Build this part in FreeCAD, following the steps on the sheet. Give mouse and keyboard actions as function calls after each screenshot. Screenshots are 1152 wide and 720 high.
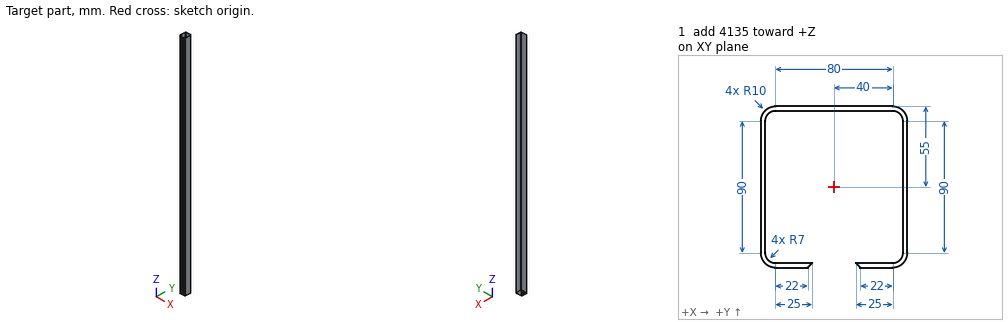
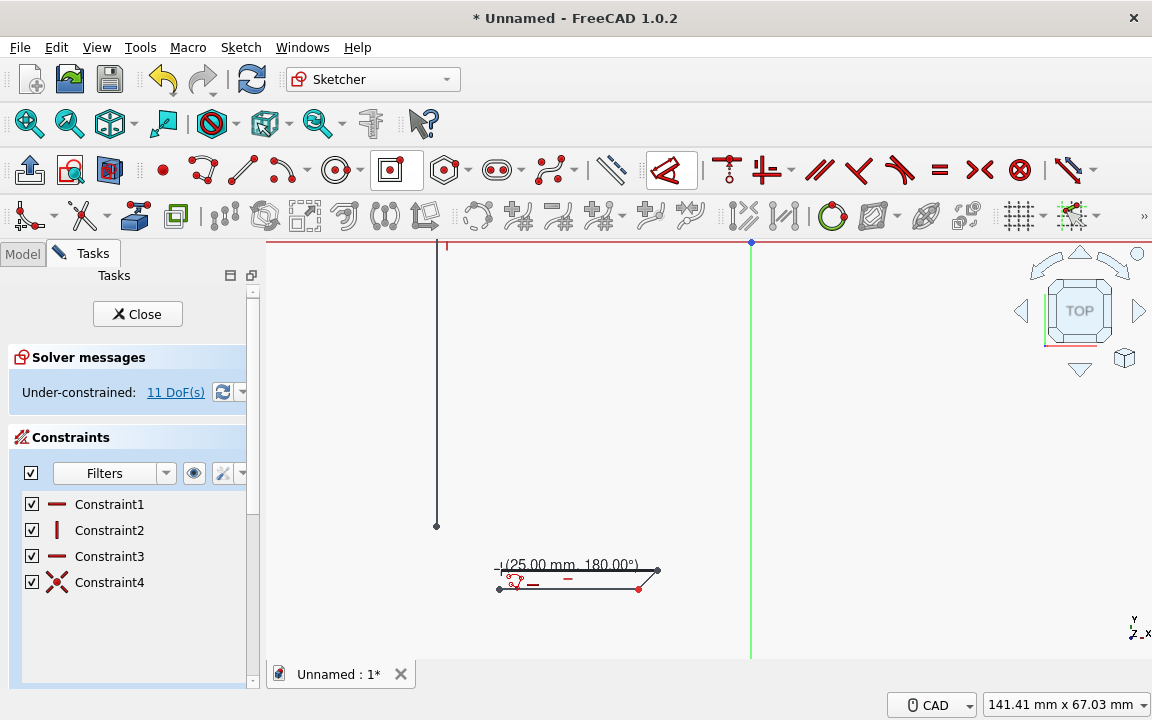
click(500, 569)
right_click(500, 569)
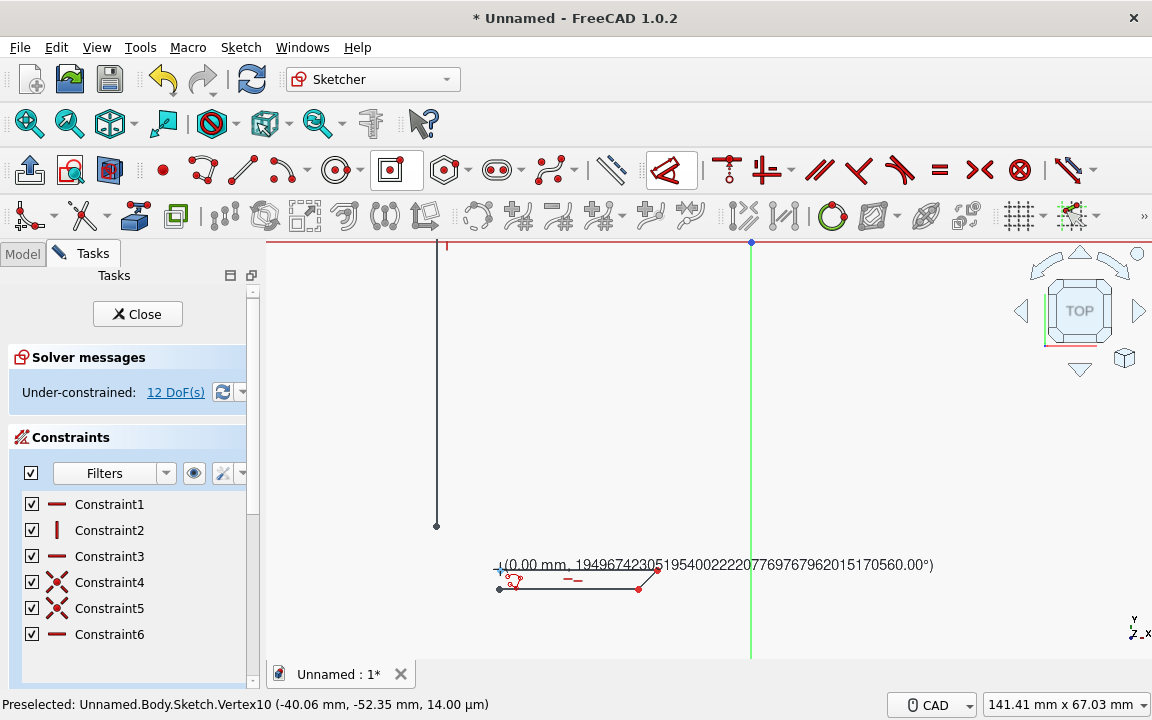
click(244, 170)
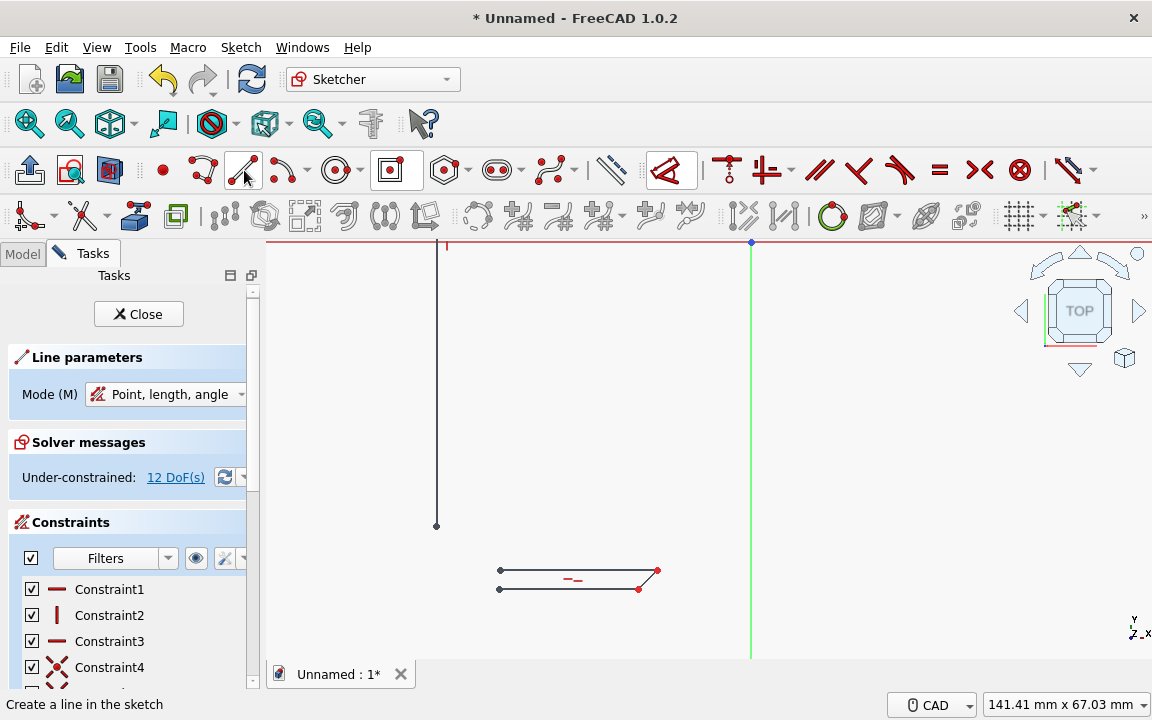
click(457, 524)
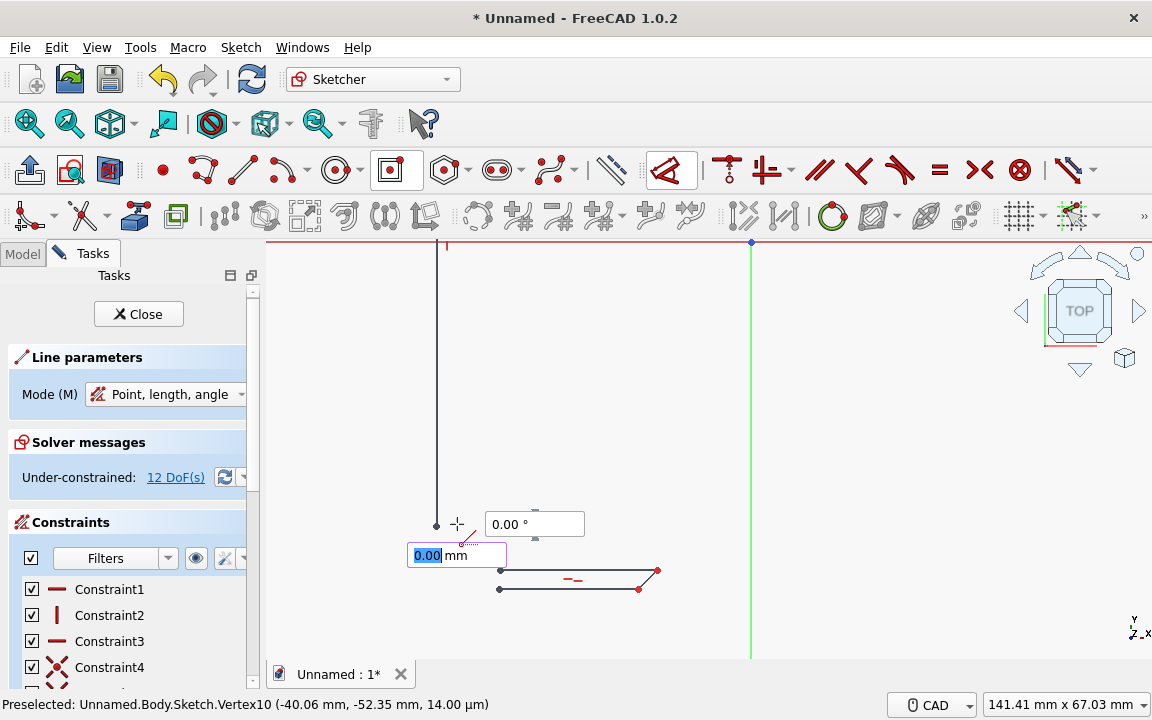
scroll(576, 569, down, 5)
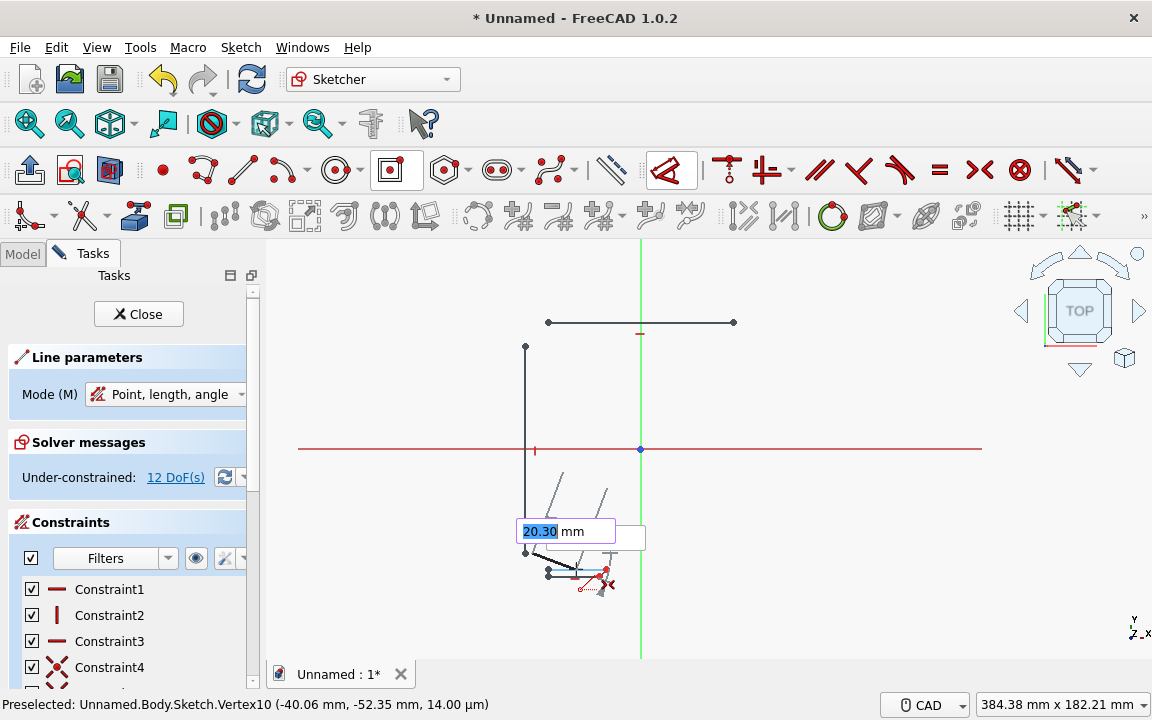
scroll(532, 346, up, 5)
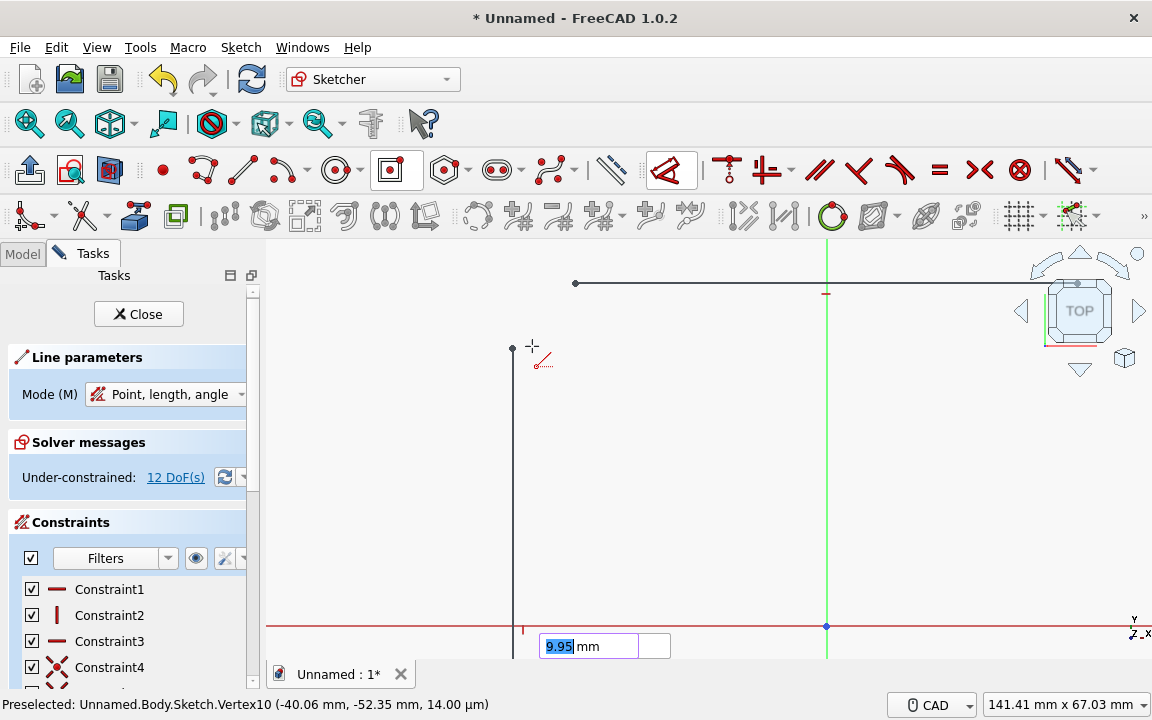
click(533, 344)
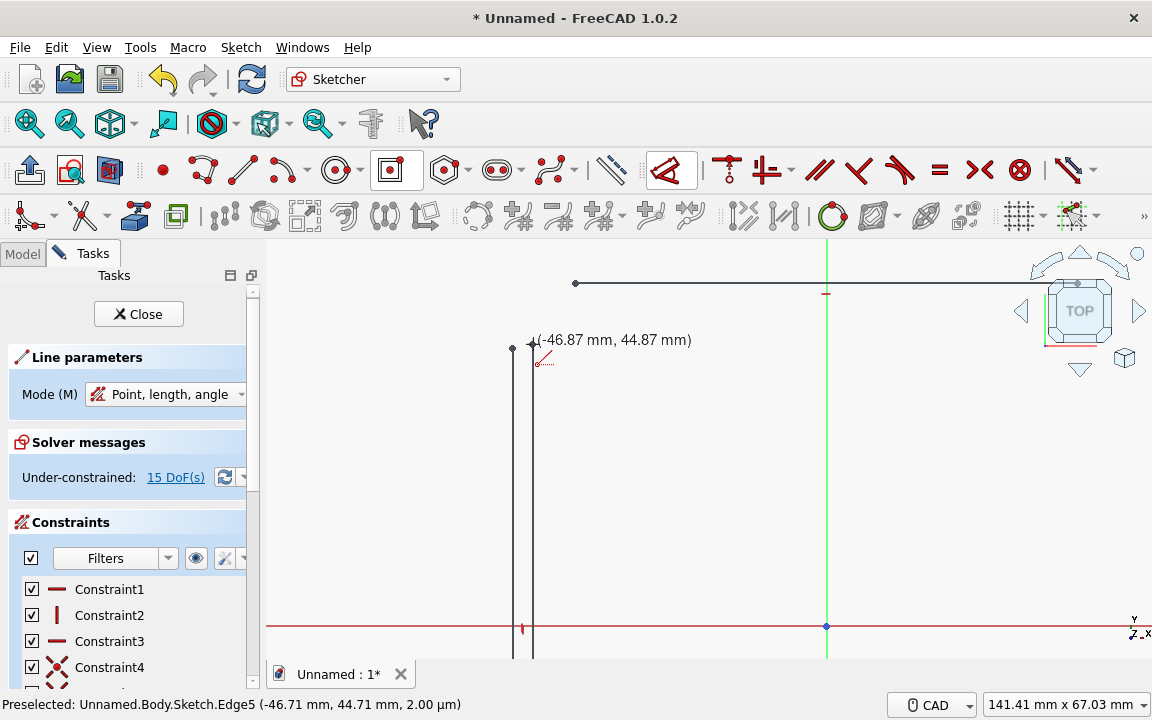
click(576, 300)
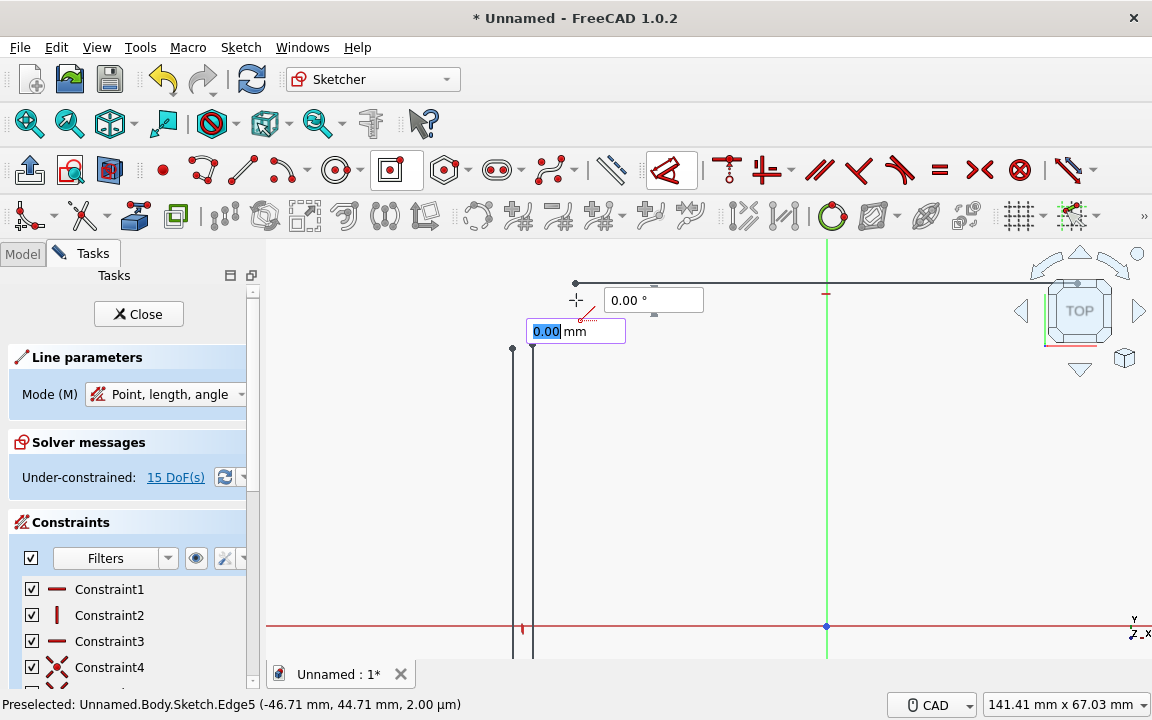
scroll(532, 346, down, 5)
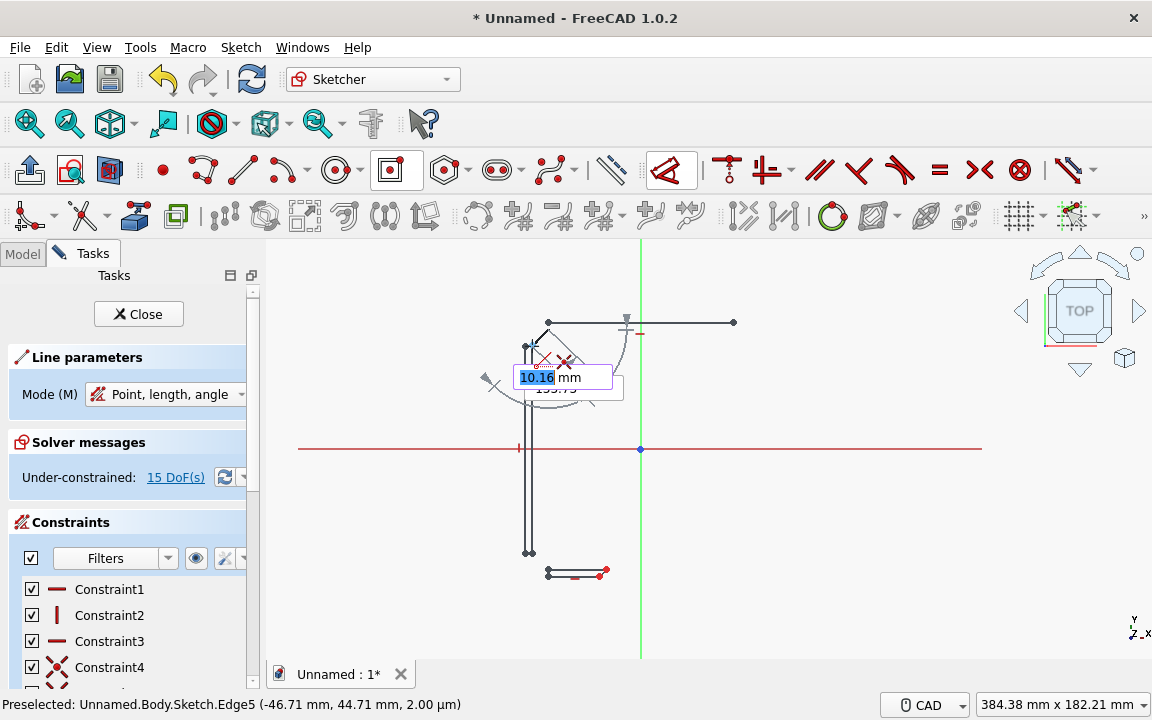
scroll(733, 329, up, 5)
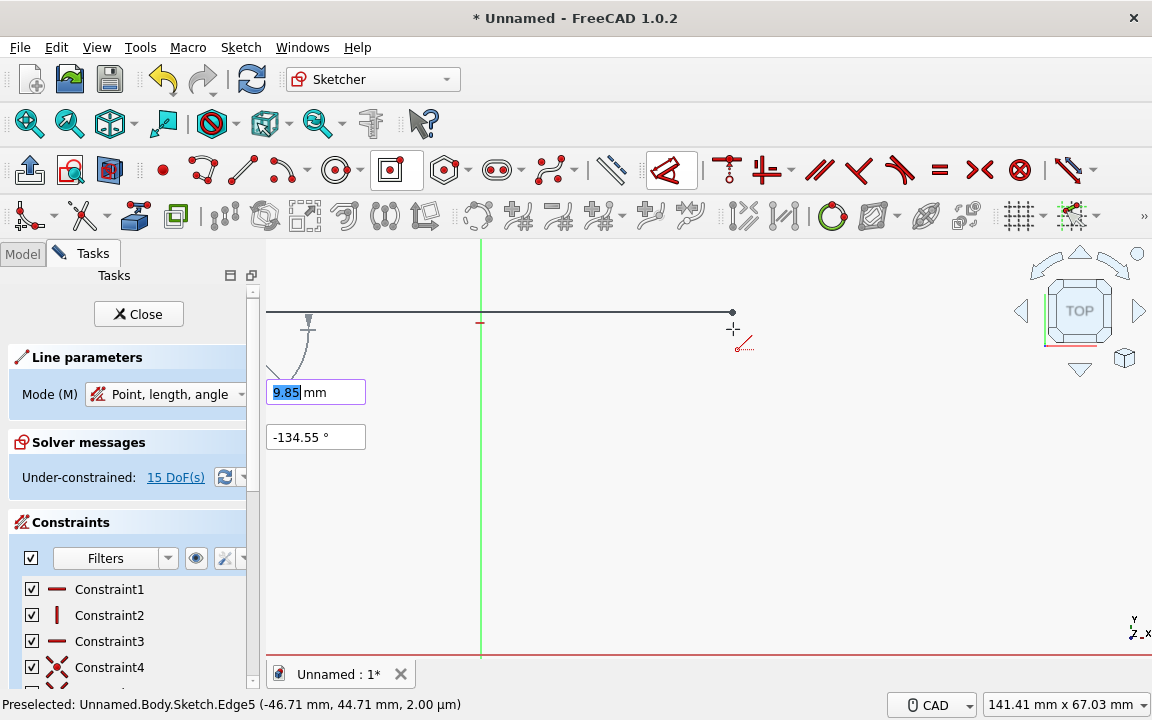
click(732, 329)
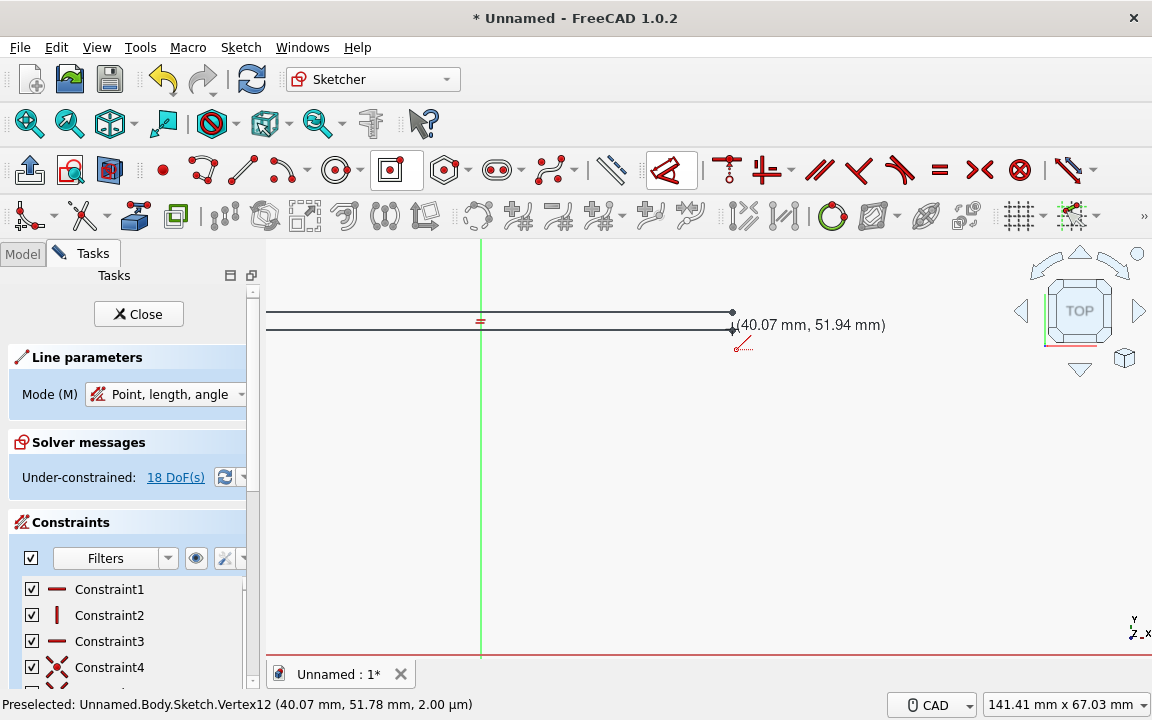
click(775, 373)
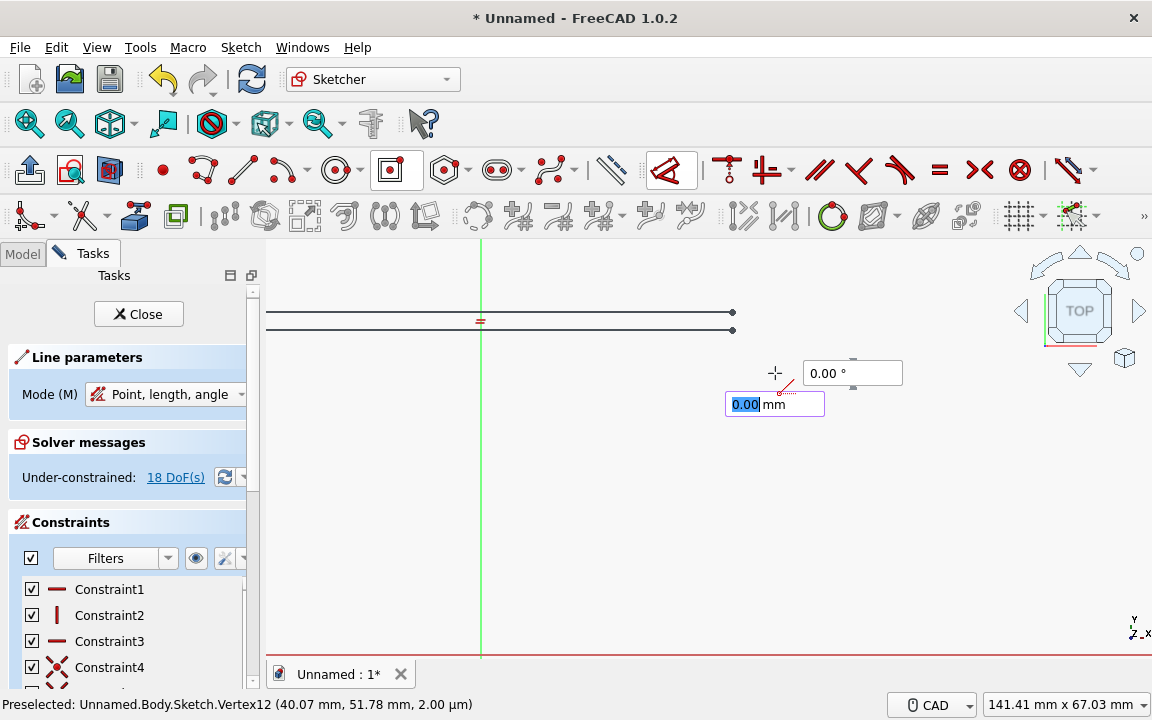
scroll(733, 329, down, 5)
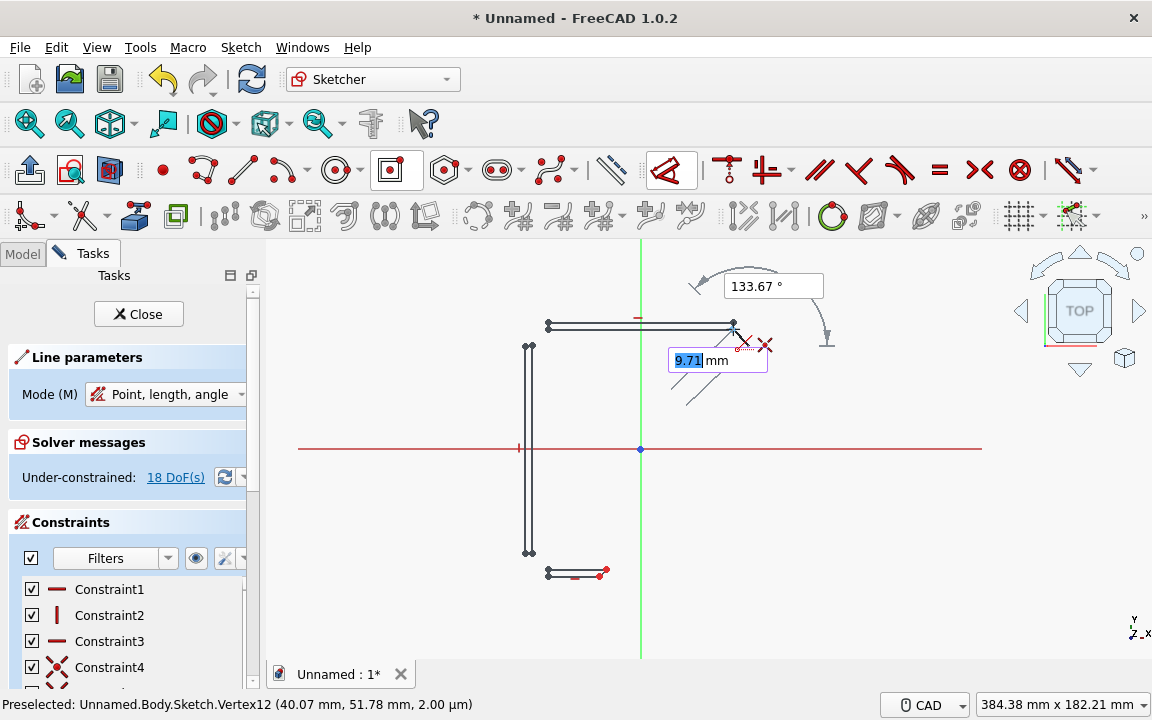
click(749, 553)